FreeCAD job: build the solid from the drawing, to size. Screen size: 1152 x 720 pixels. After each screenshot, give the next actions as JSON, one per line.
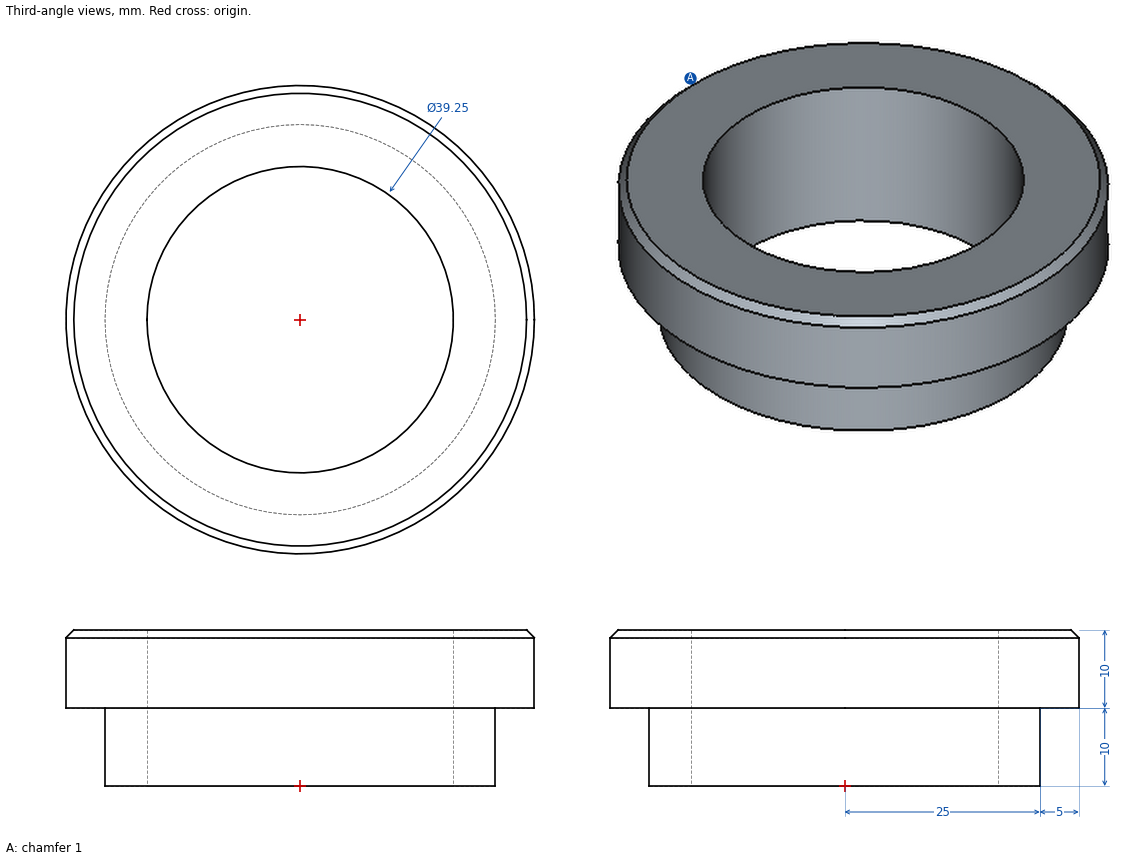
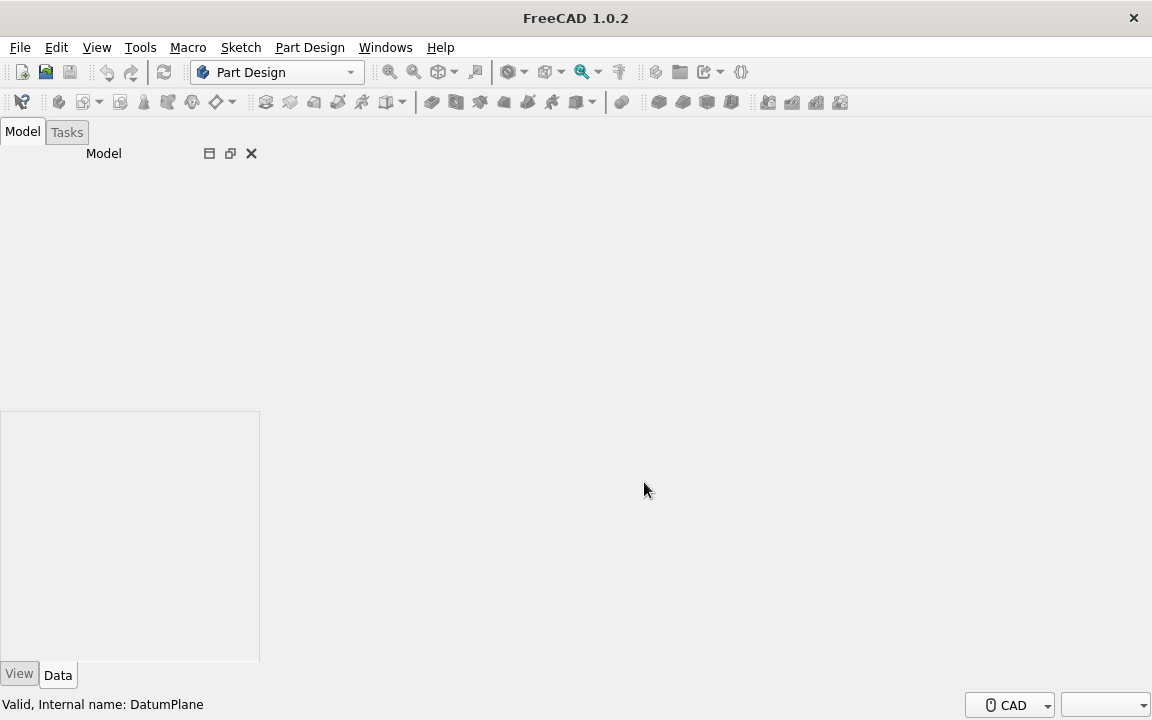
{"action": "left_click", "coordinate": [22, 72]}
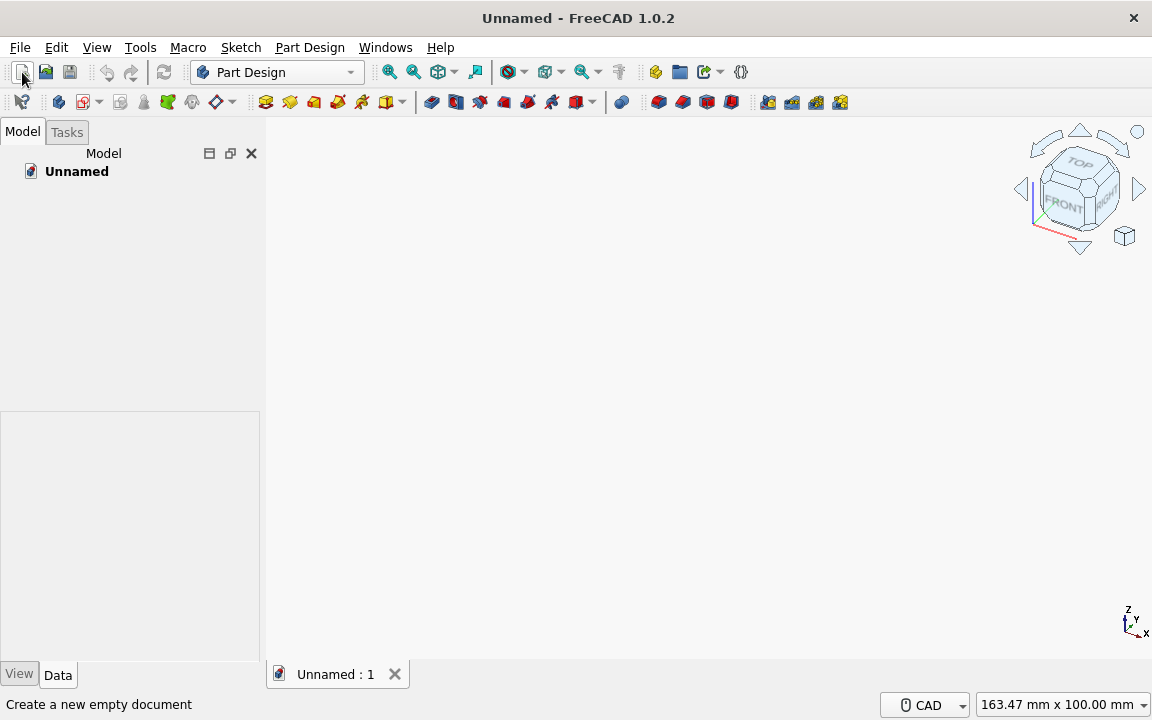
{"action": "left_click", "coordinate": [84, 102]}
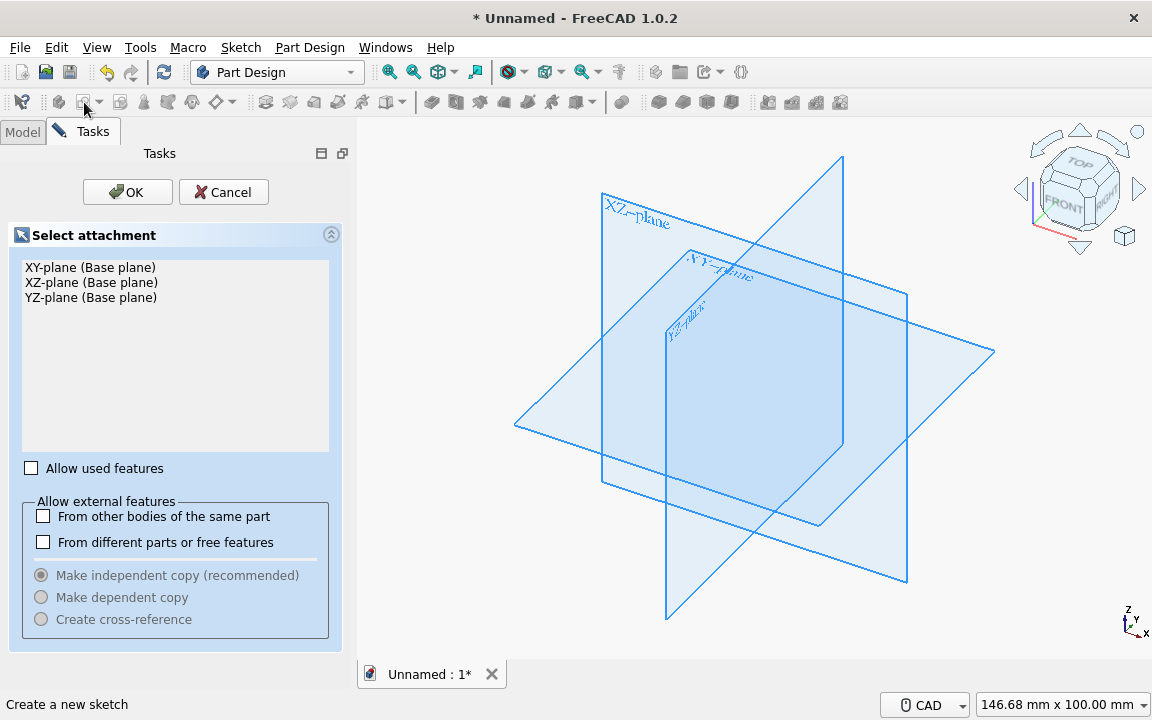
{"action": "left_click", "coordinate": [82, 298]}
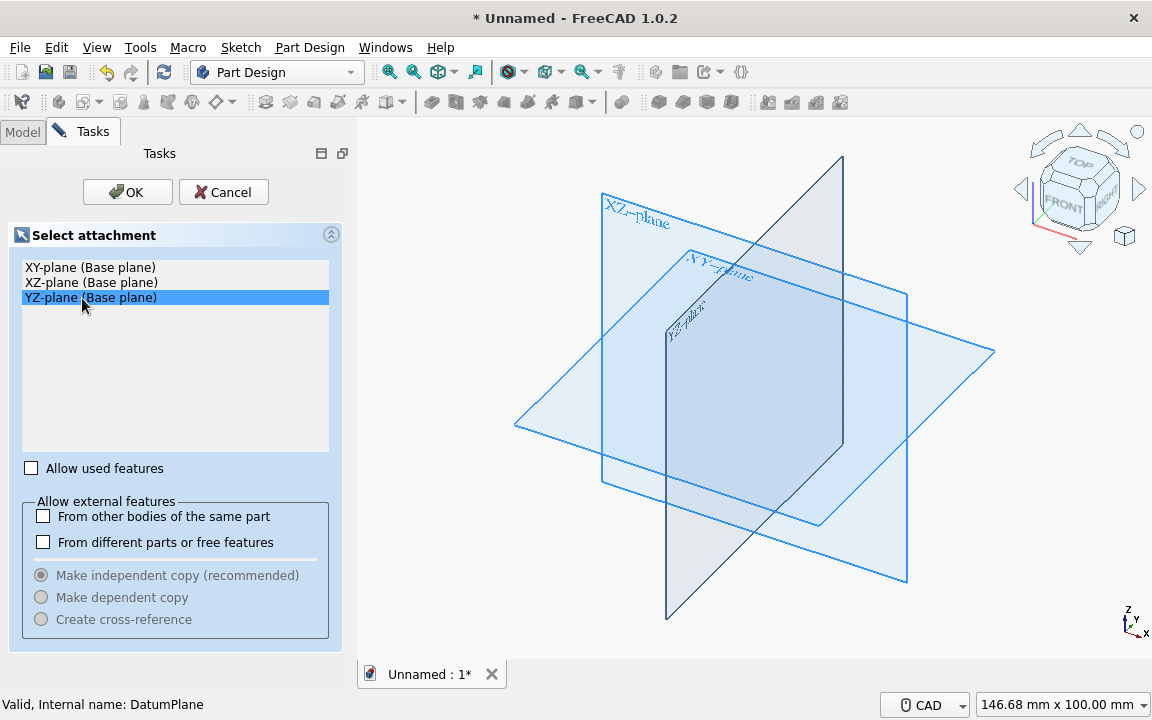
{"action": "left_click", "coordinate": [128, 192]}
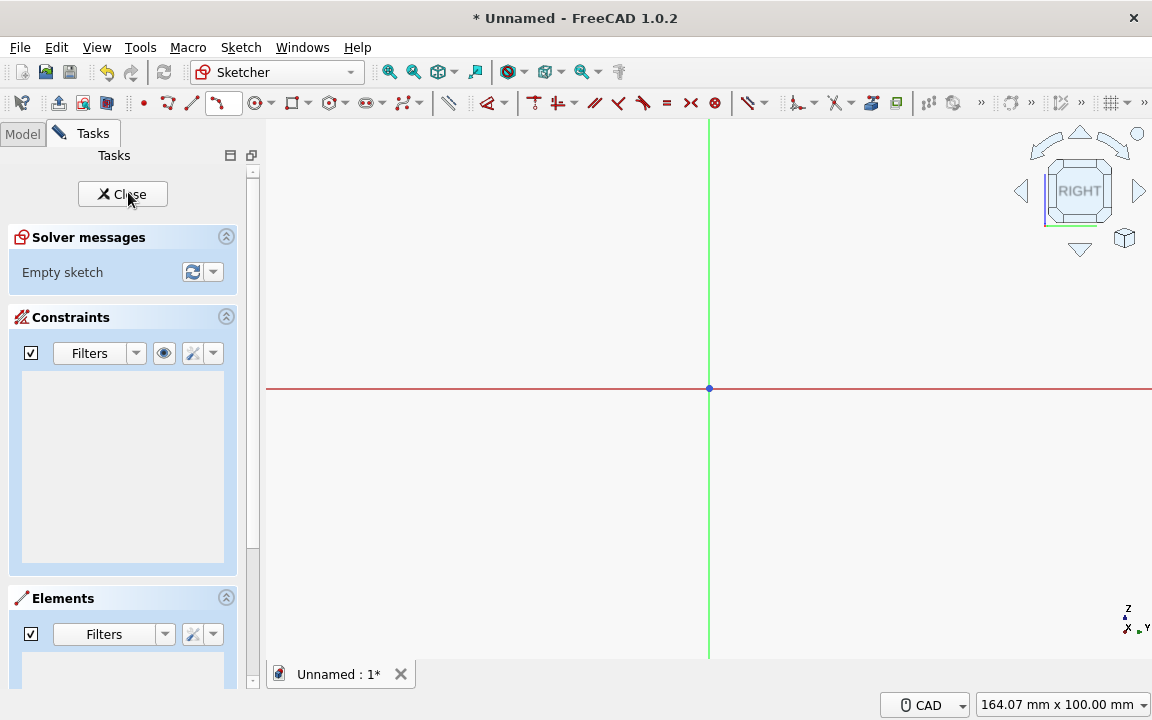
{"action": "scroll", "coordinate": [854, 312], "scroll_direction": "up", "scroll_amount": 6}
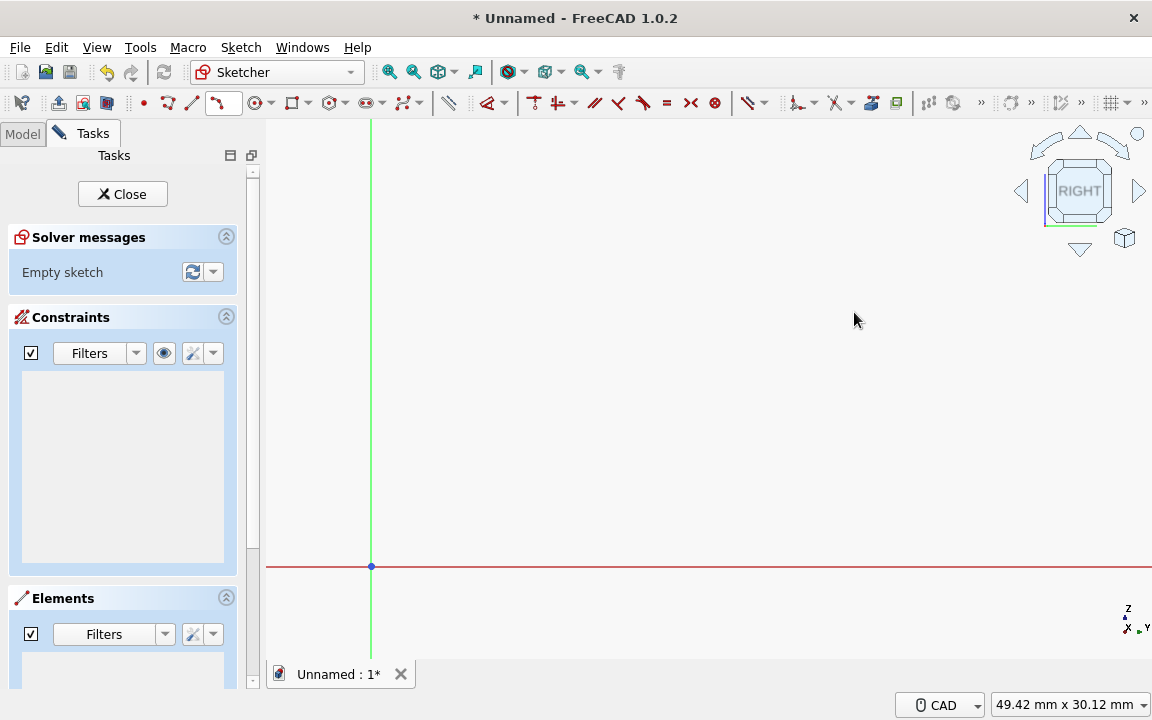
{"action": "left_click", "coordinate": [168, 104]}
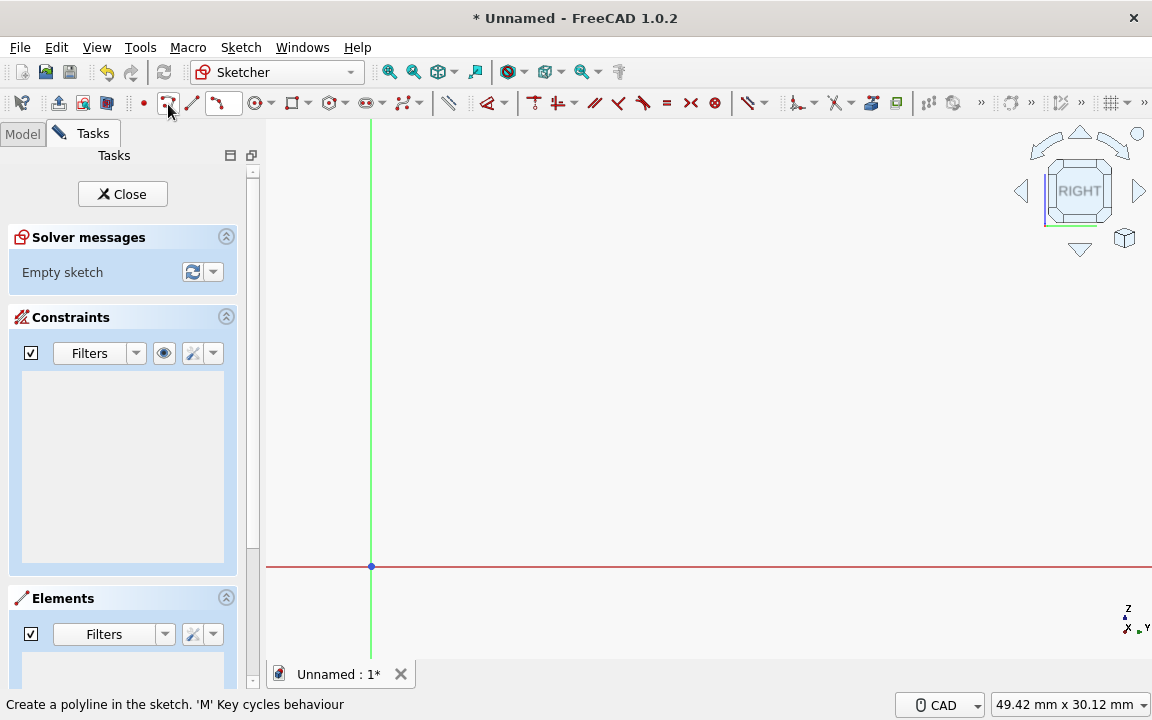
{"action": "left_click", "coordinate": [371, 567]}
{"action": "left_click", "coordinate": [819, 558]}
{"action": "left_click", "coordinate": [819, 388]}
{"action": "left_click", "coordinate": [909, 388]}
{"action": "left_click", "coordinate": [909, 208]}
{"action": "left_click", "coordinate": [380, 208]}
{"action": "left_click", "coordinate": [371, 567]}
{"action": "key", "text": "Escape"}
{"action": "key", "text": "Escape"}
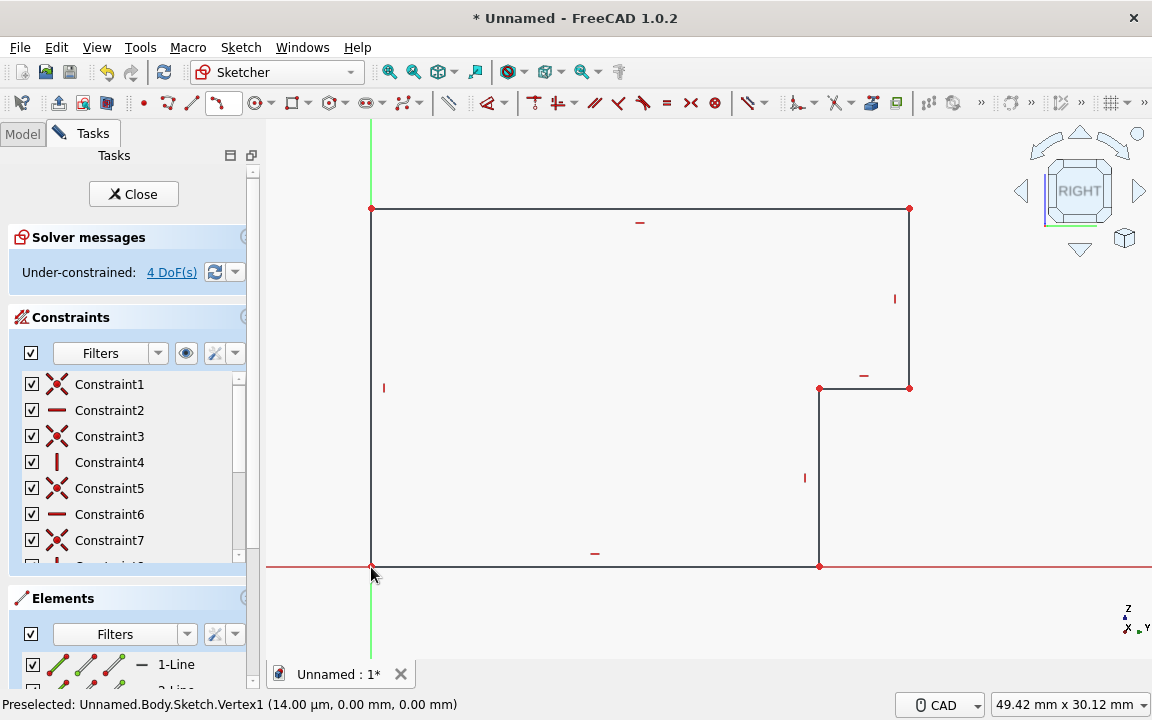
{"action": "left_click", "coordinate": [488, 104]}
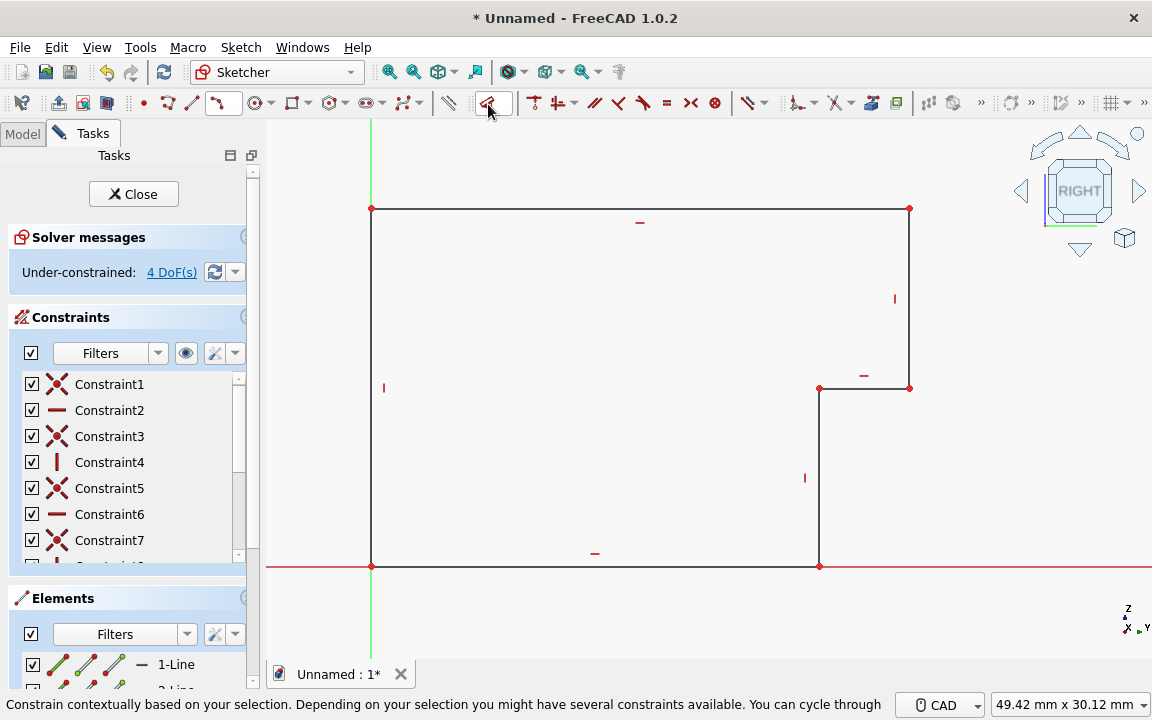
{"action": "left_click", "coordinate": [846, 389]}
{"action": "left_click", "coordinate": [864, 423]}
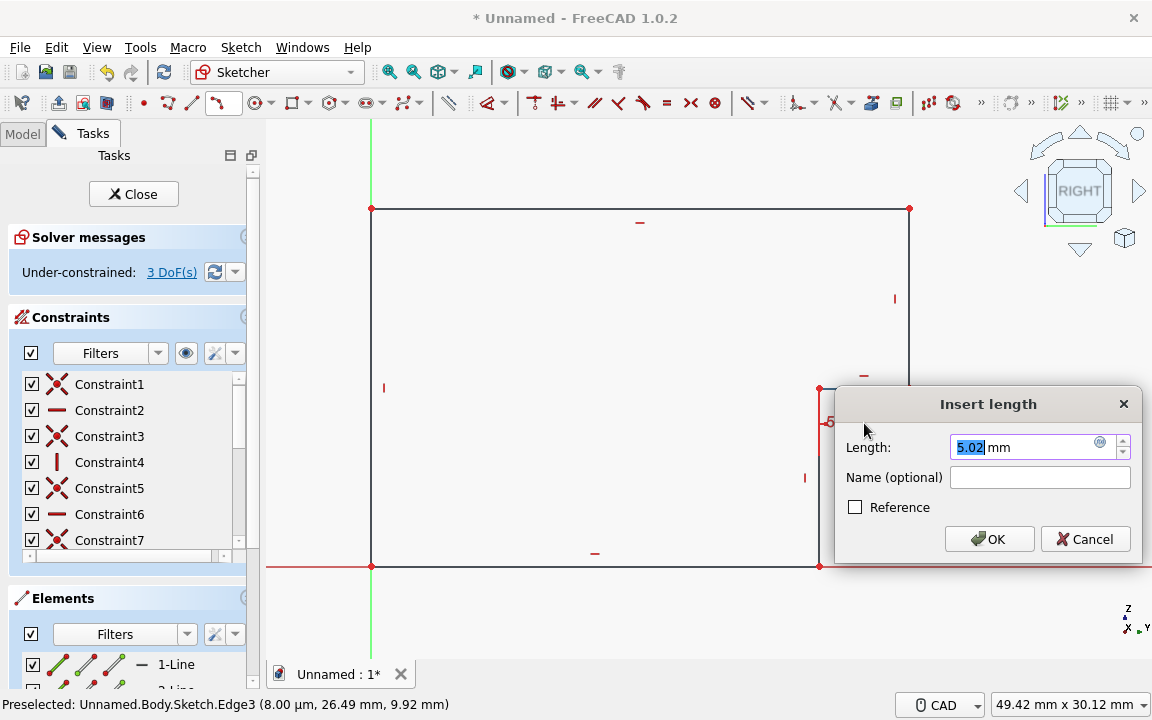
{"action": "type", "text": "5"}
{"action": "key", "text": "Return"}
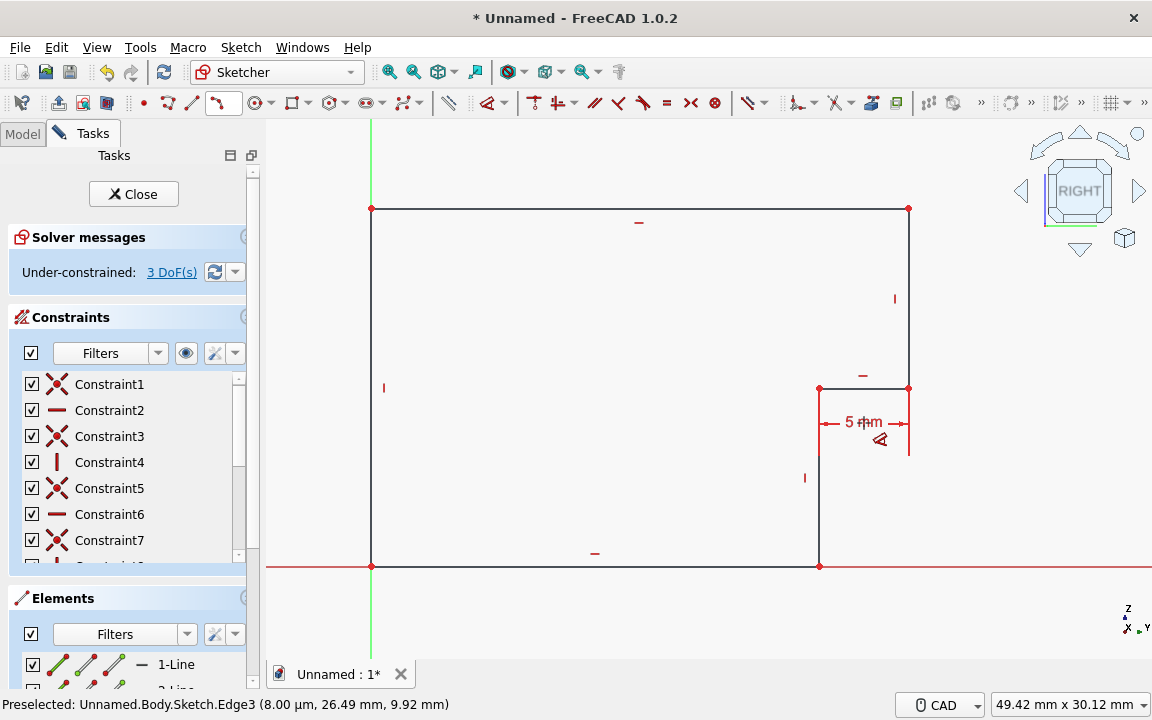
{"action": "left_click", "coordinate": [505, 567]}
{"action": "left_click", "coordinate": [595, 601]}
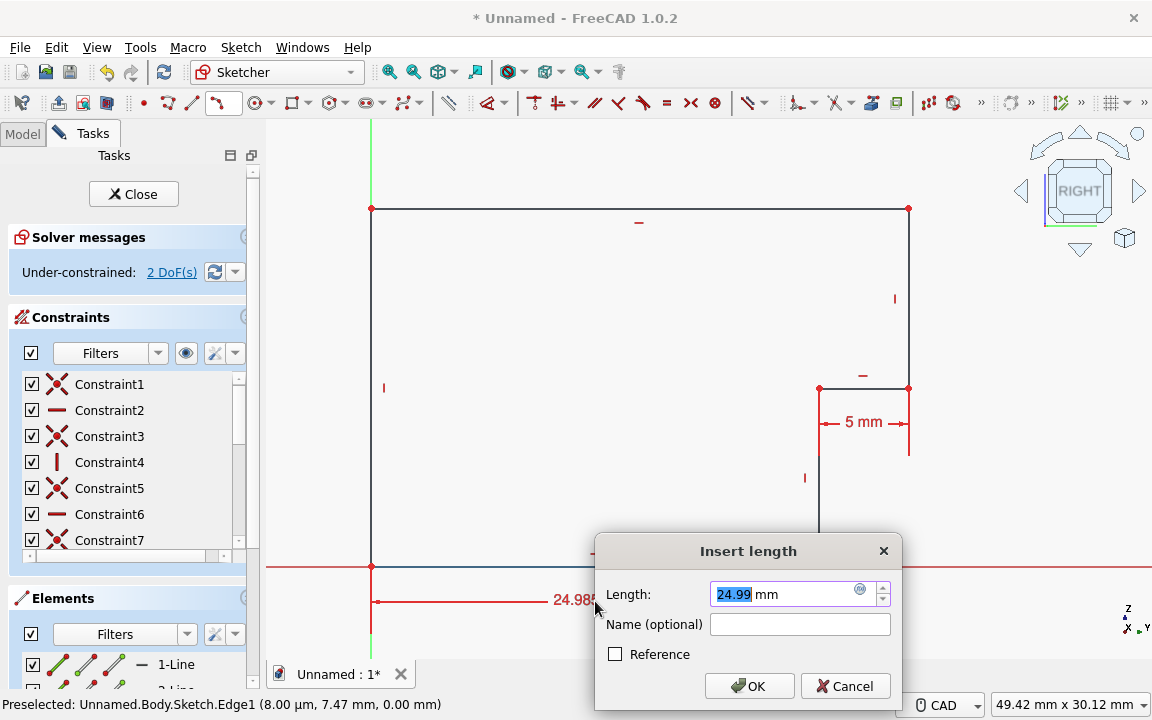
{"action": "type", "text": "25"}
{"action": "key", "text": "Return"}